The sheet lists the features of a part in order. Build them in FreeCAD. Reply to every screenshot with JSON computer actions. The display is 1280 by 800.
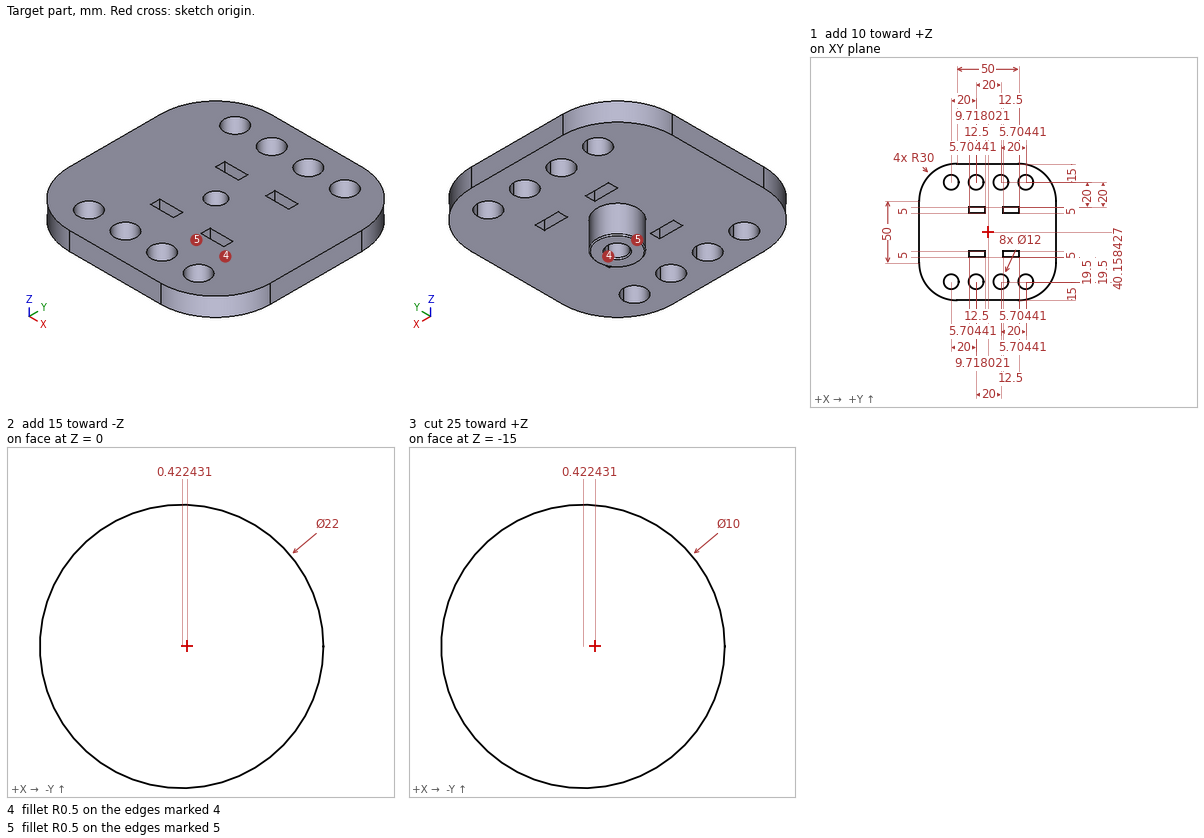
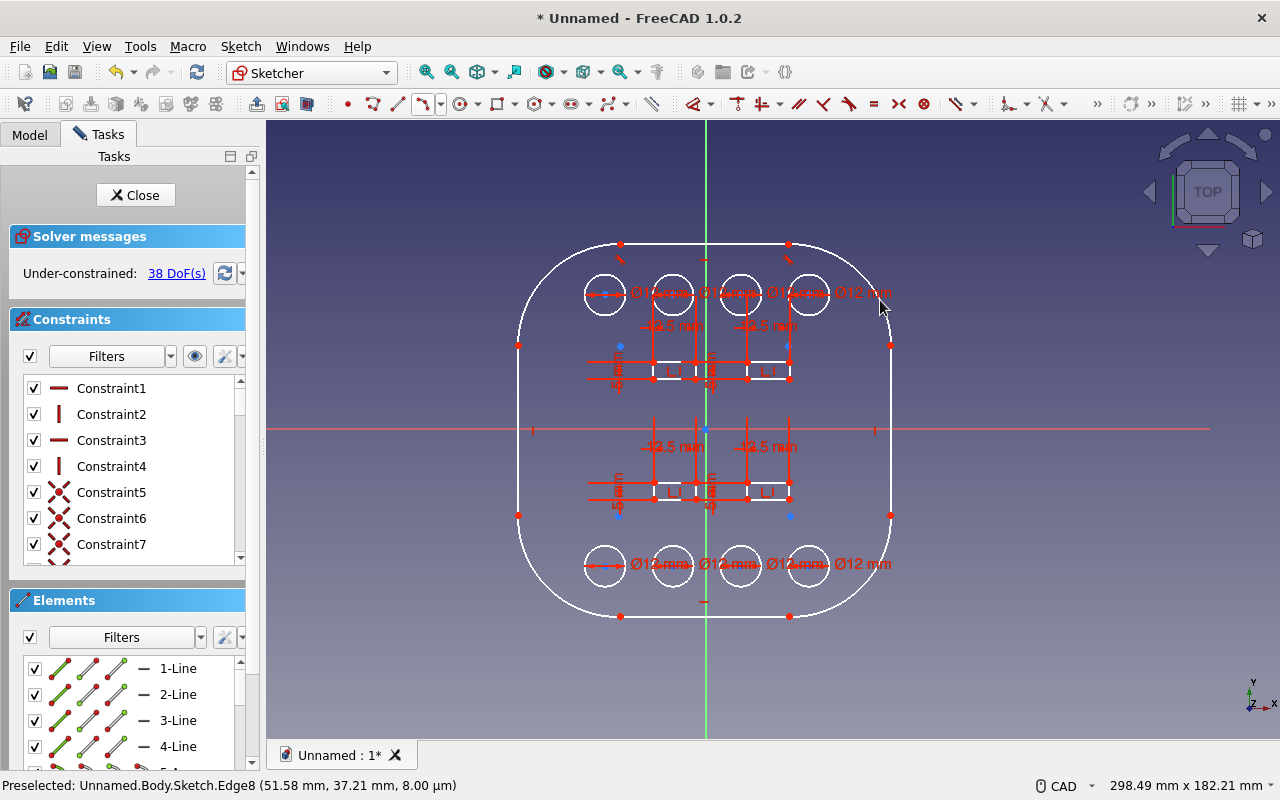
{"action": "left_click", "coordinate": [518, 397]}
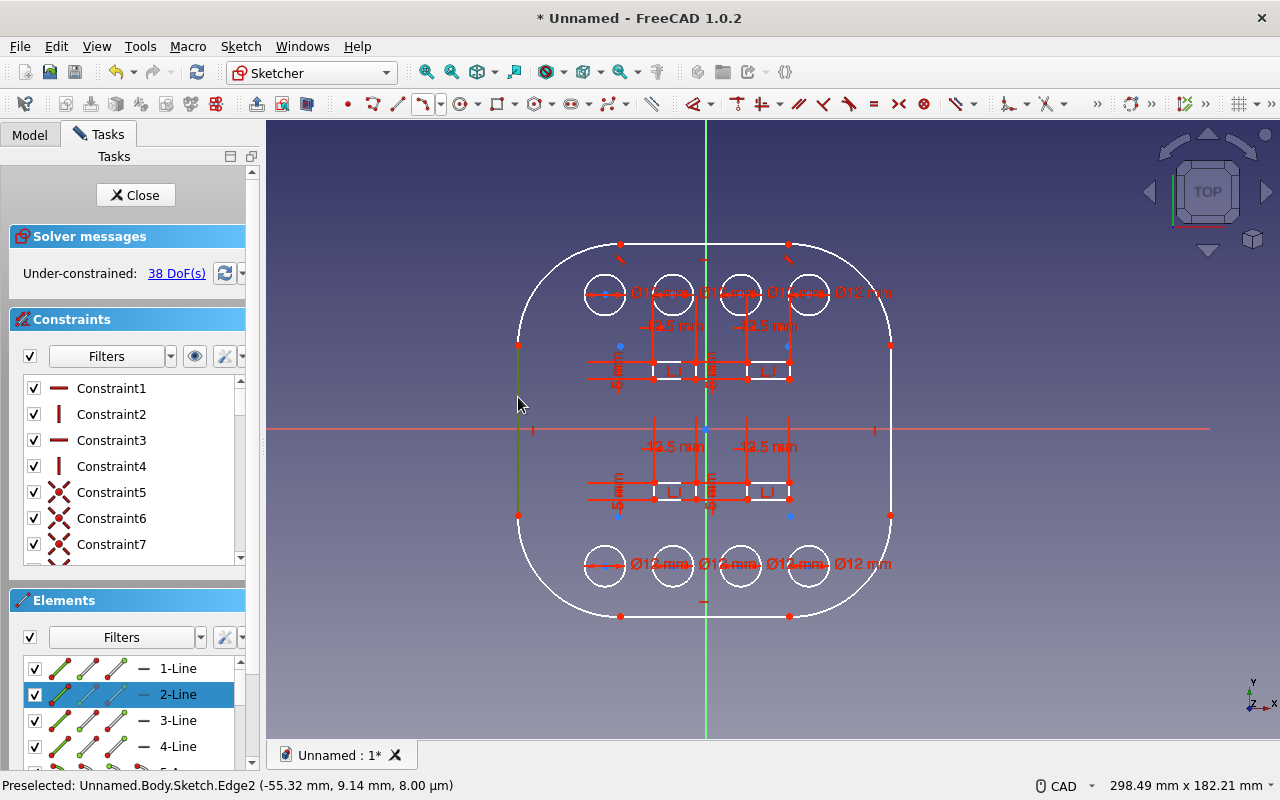
{"action": "left_click", "coordinate": [574, 255]}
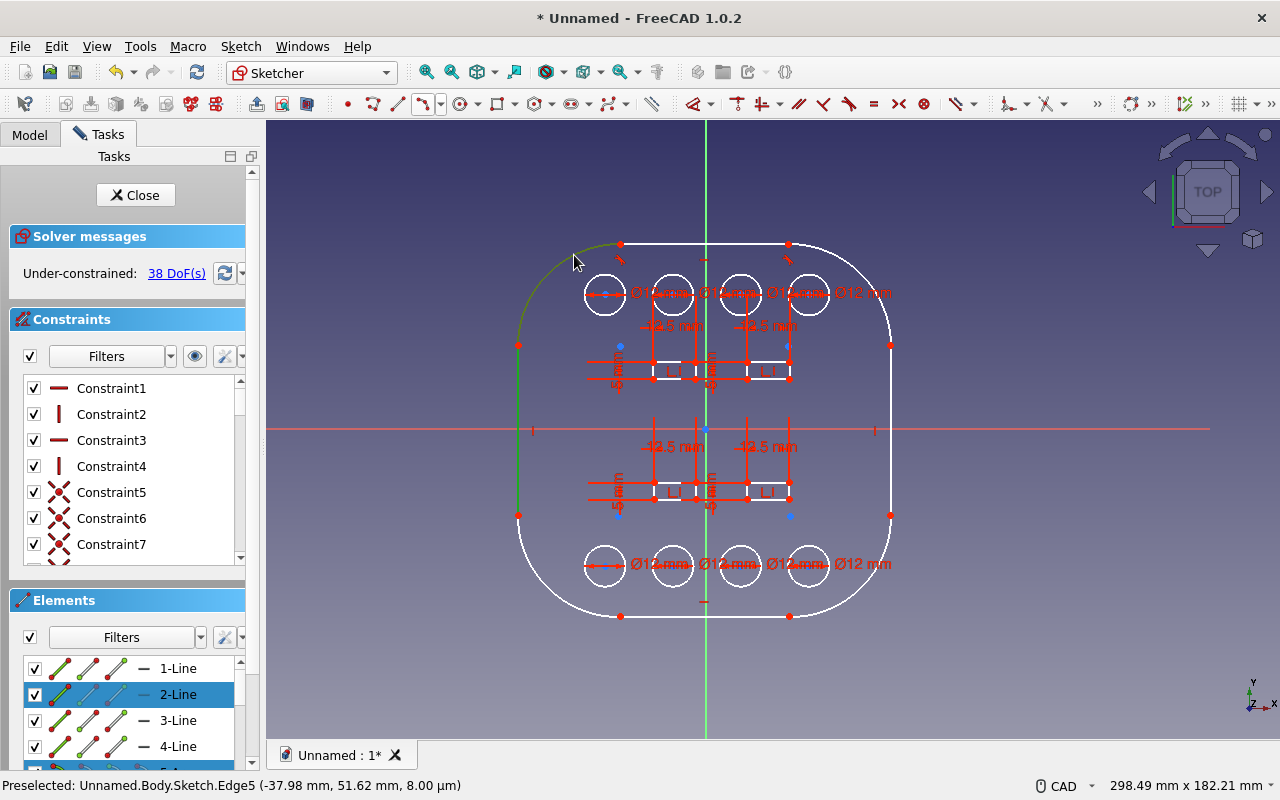
{"action": "left_click", "coordinate": [849, 104]}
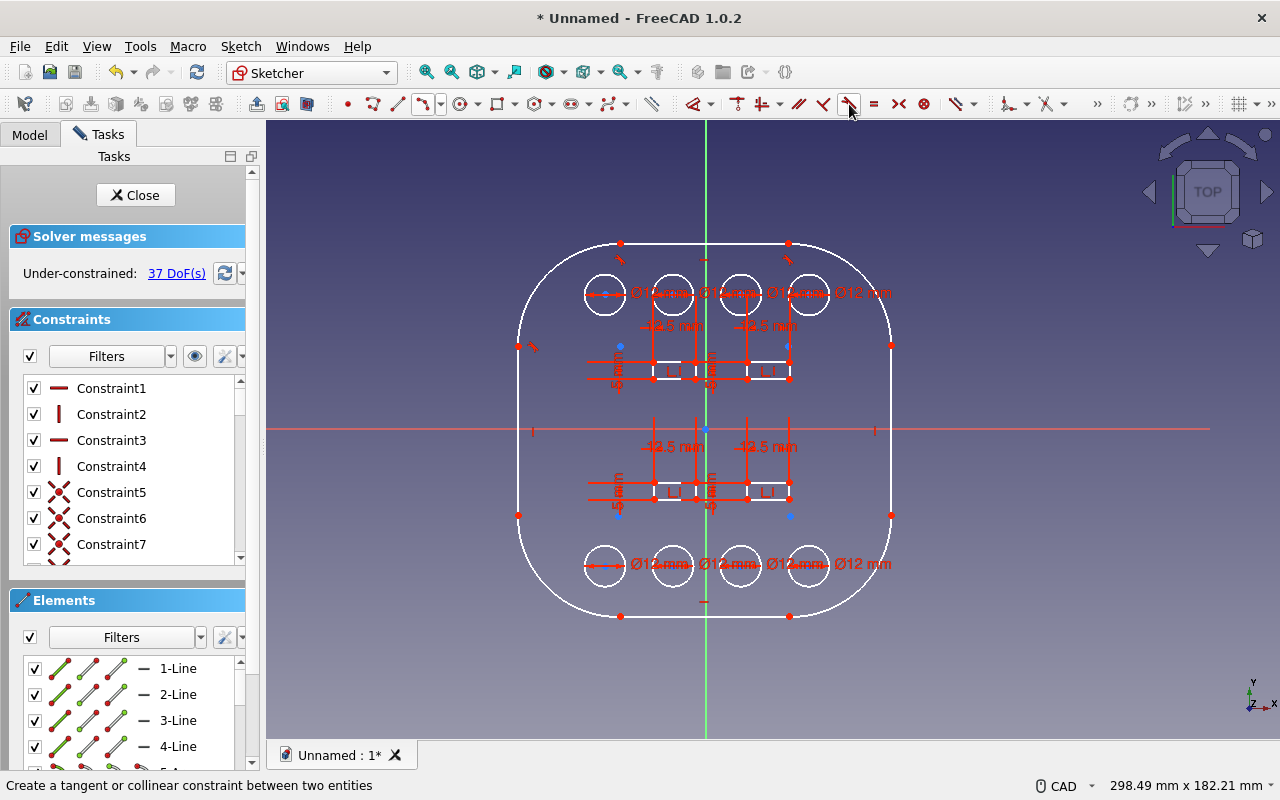
{"action": "left_click", "coordinate": [518, 397]}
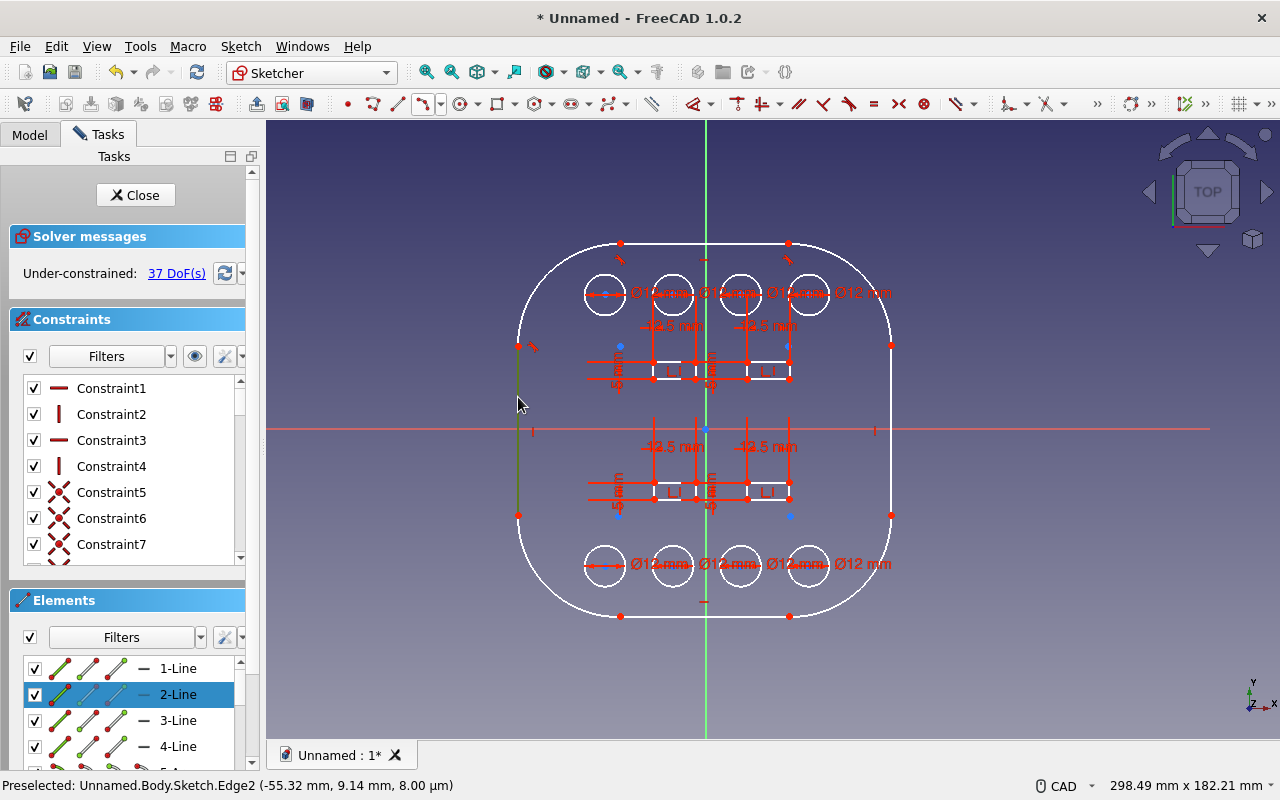
{"action": "left_click", "coordinate": [529, 562]}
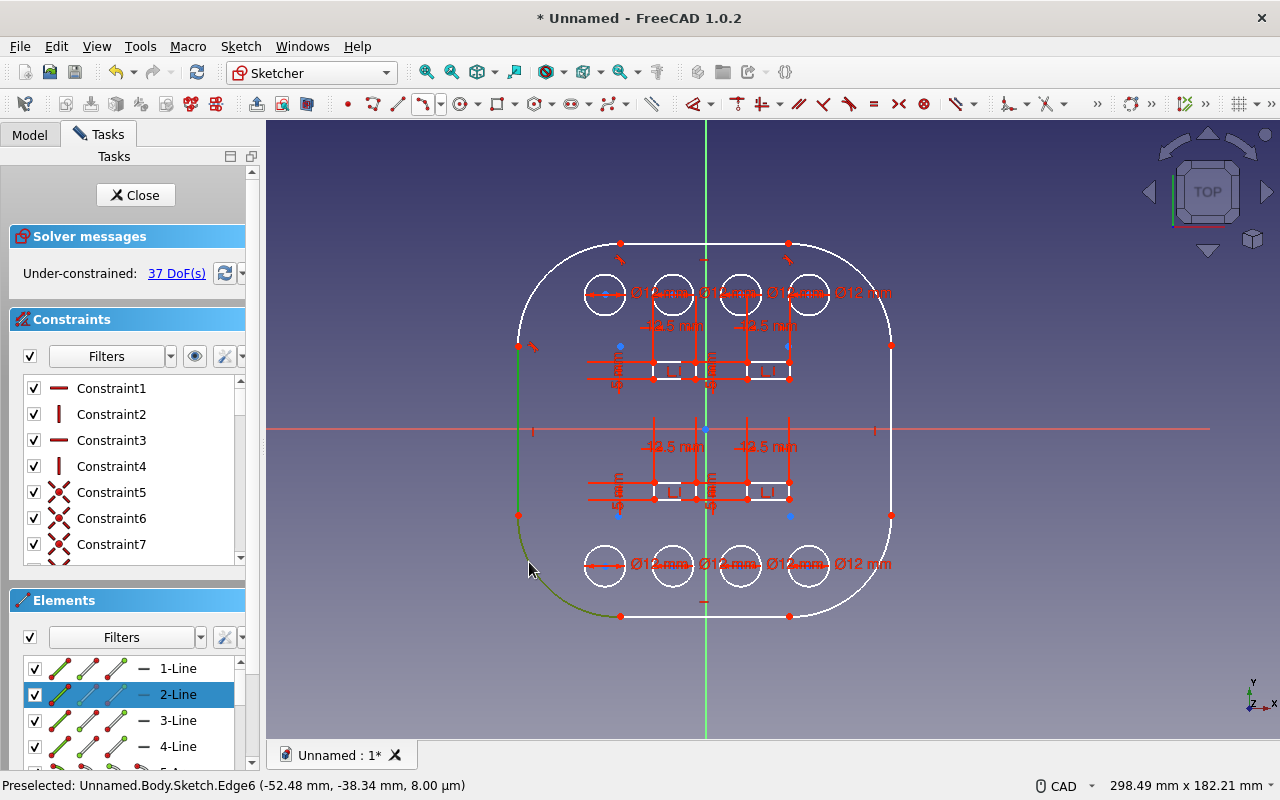
{"action": "left_click", "coordinate": [849, 104]}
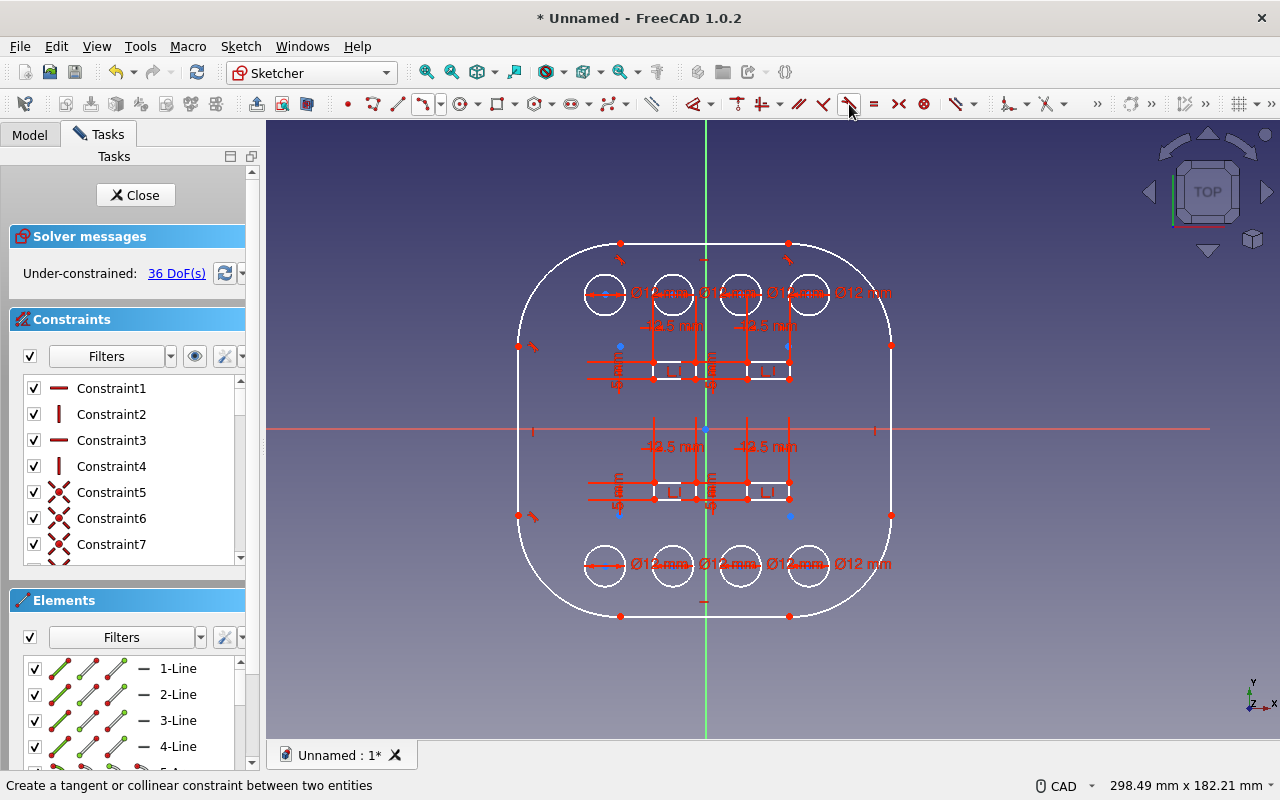
{"action": "left_click", "coordinate": [671, 617]}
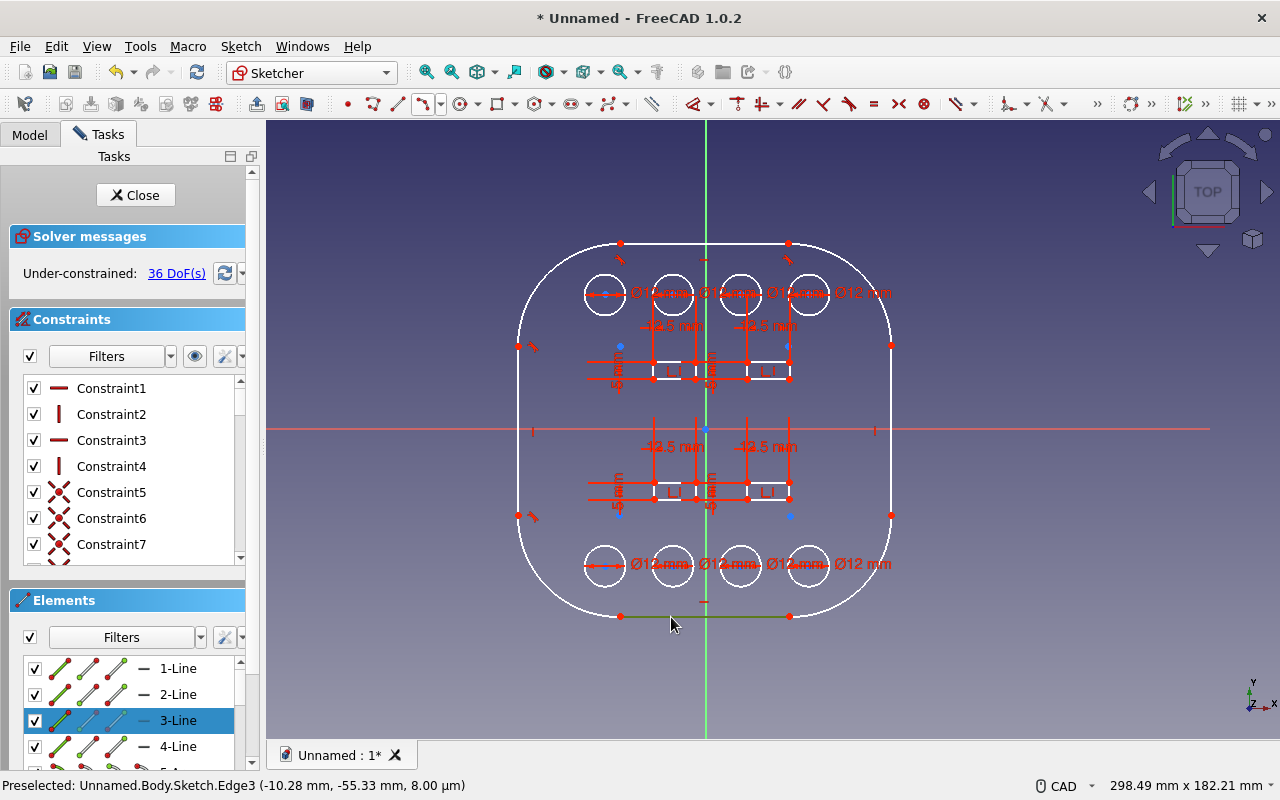
{"action": "left_click", "coordinate": [529, 562]}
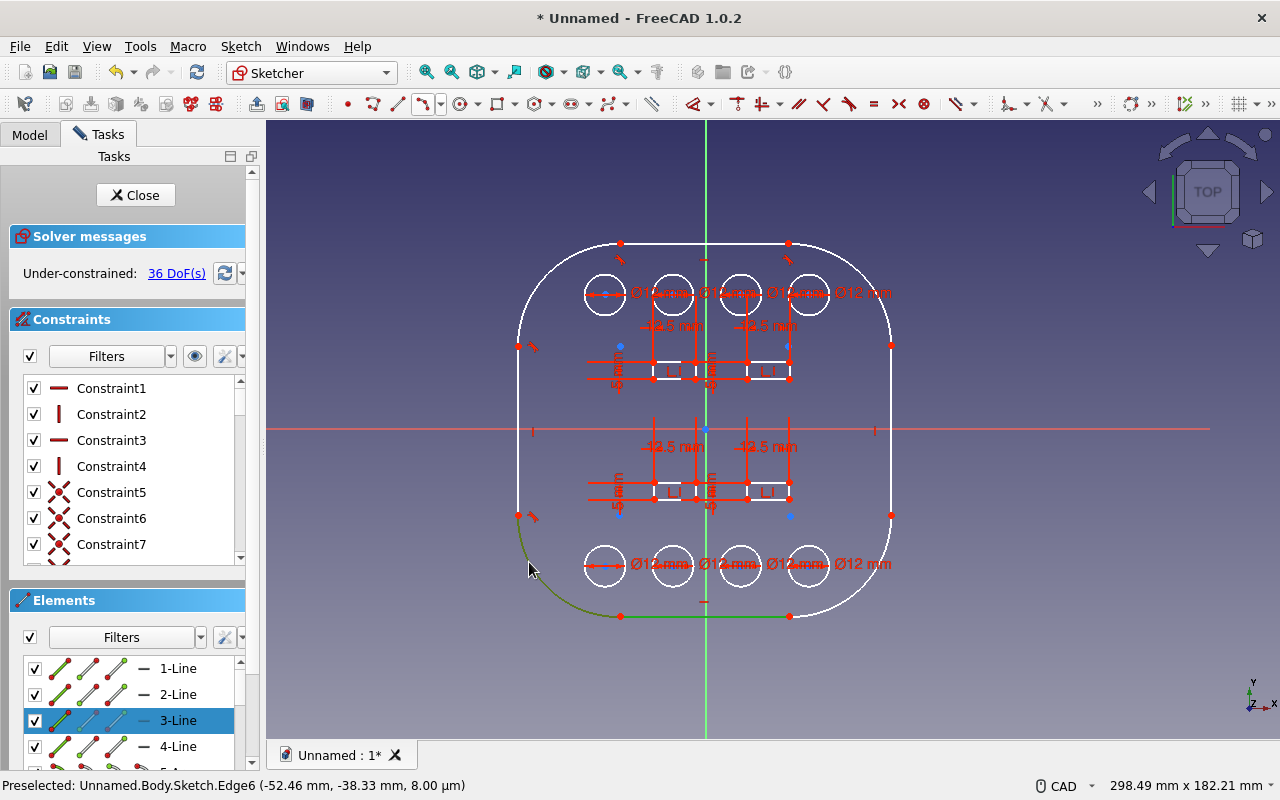
{"action": "left_click", "coordinate": [849, 104]}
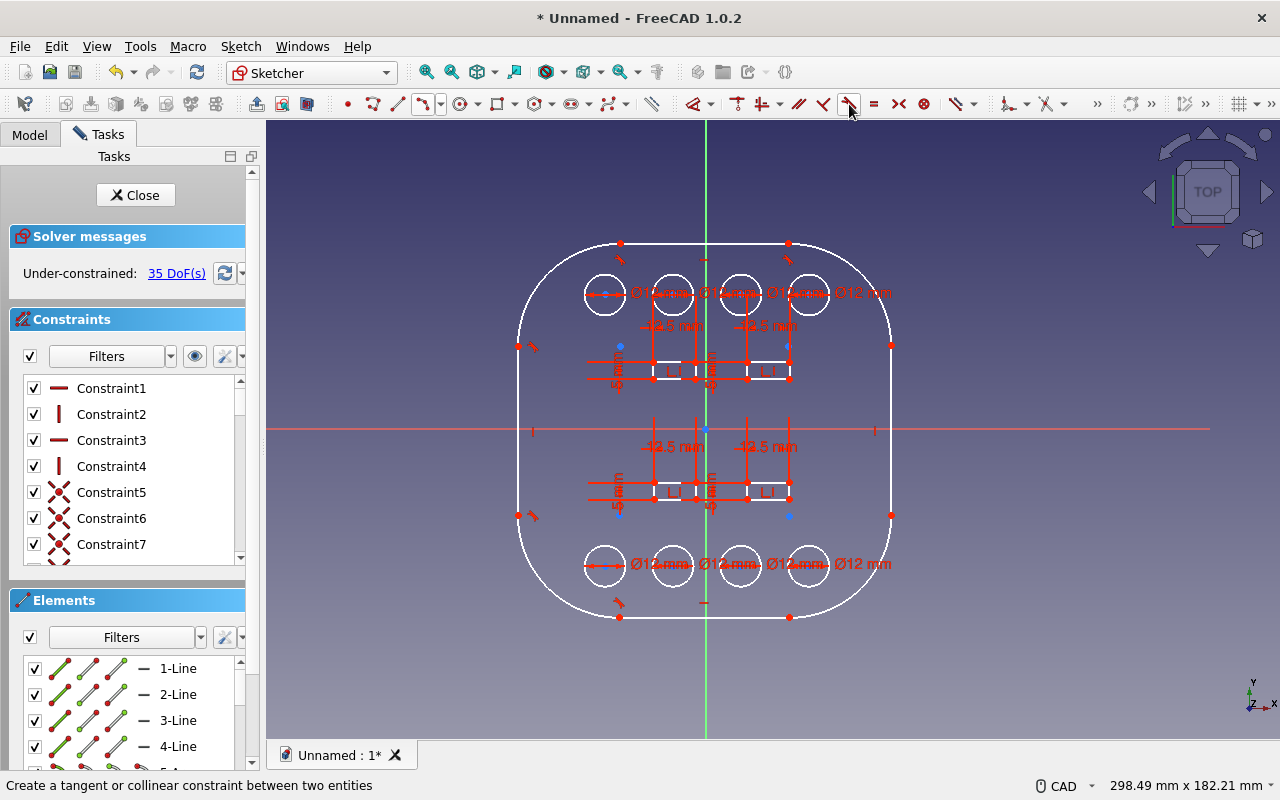
{"action": "left_click", "coordinate": [671, 618]}